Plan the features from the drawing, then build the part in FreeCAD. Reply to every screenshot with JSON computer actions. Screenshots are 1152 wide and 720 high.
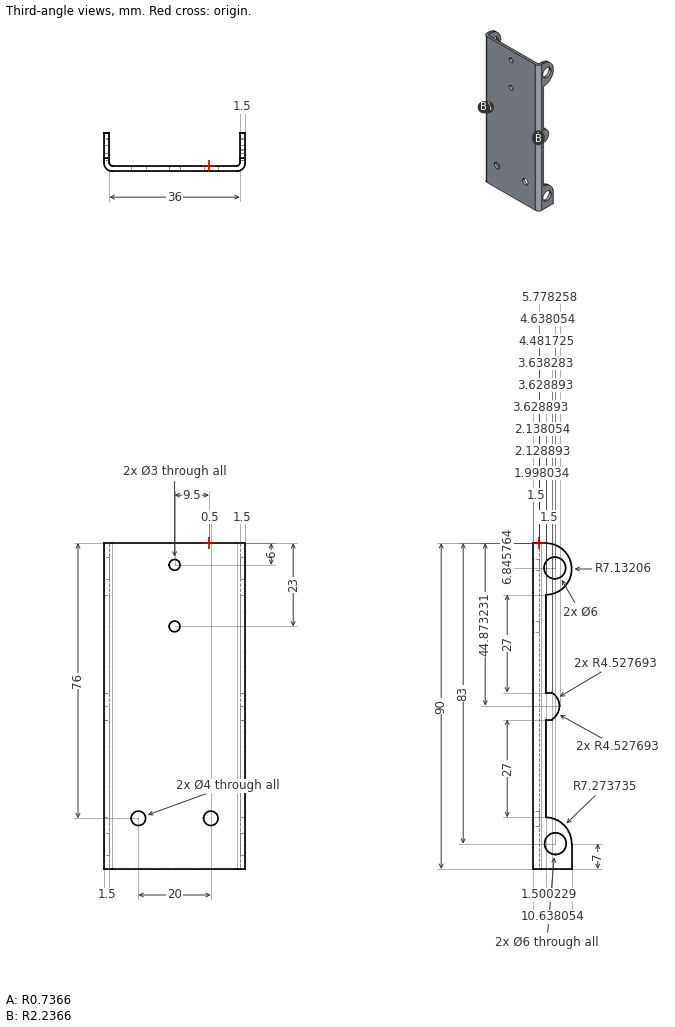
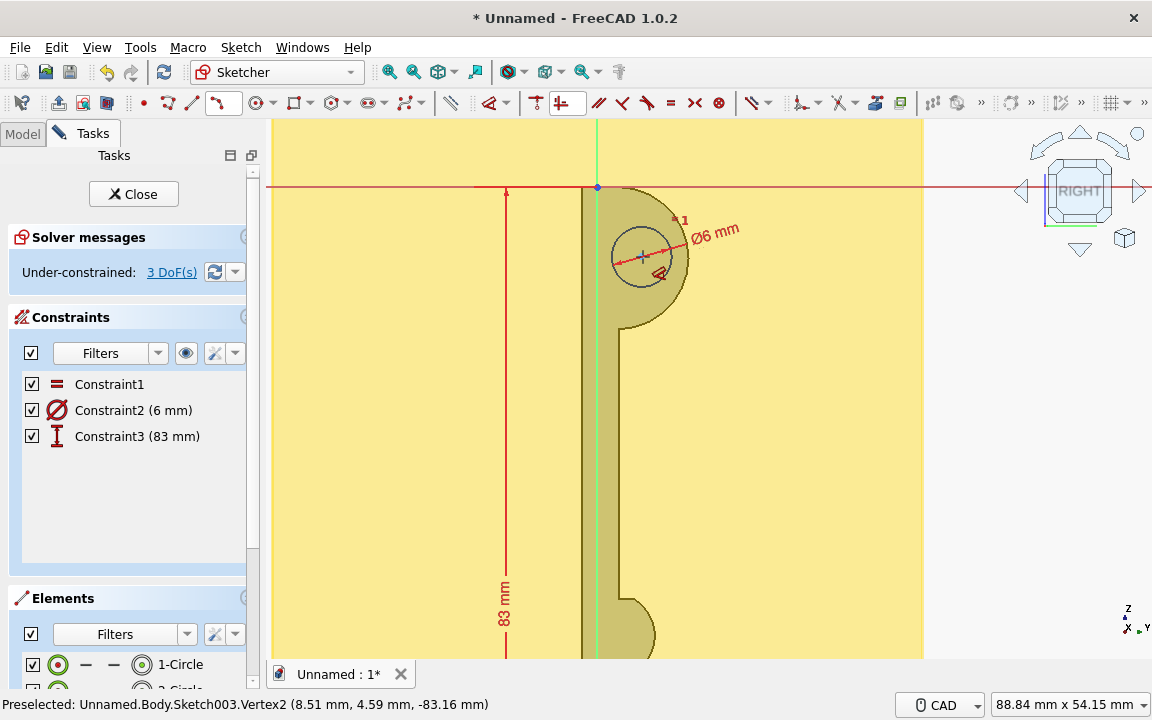
{"action": "left_click", "coordinate": [642, 257]}
{"action": "left_click", "coordinate": [620, 153]}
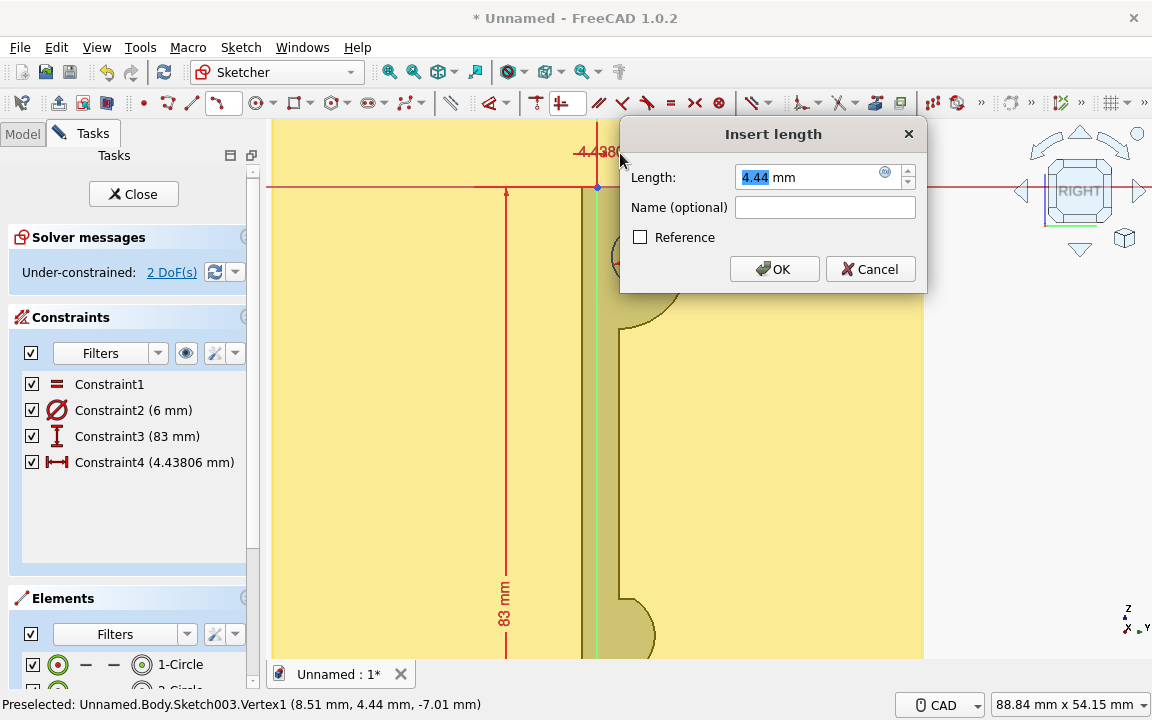
{"action": "type", "text": "4.481725"}
{"action": "key", "text": "Return"}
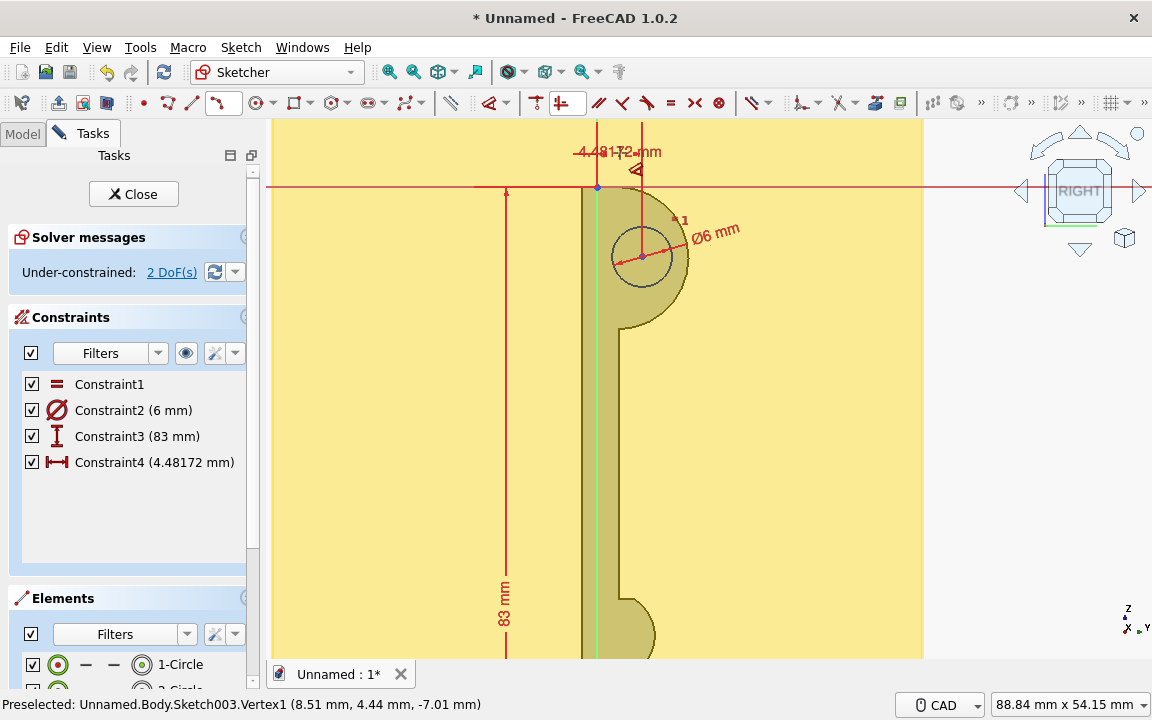
{"action": "left_click", "coordinate": [642, 257]}
{"action": "left_click", "coordinate": [563, 222]}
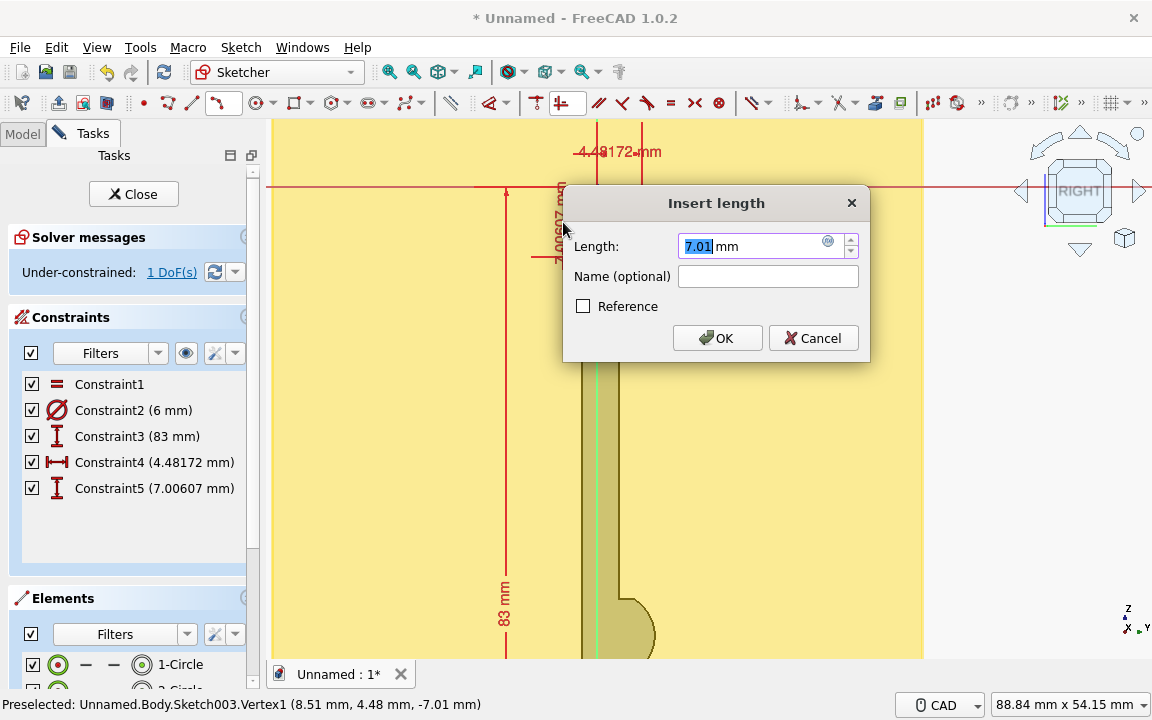
{"action": "type", "text": "6.845764"}
{"action": "key", "text": "Return"}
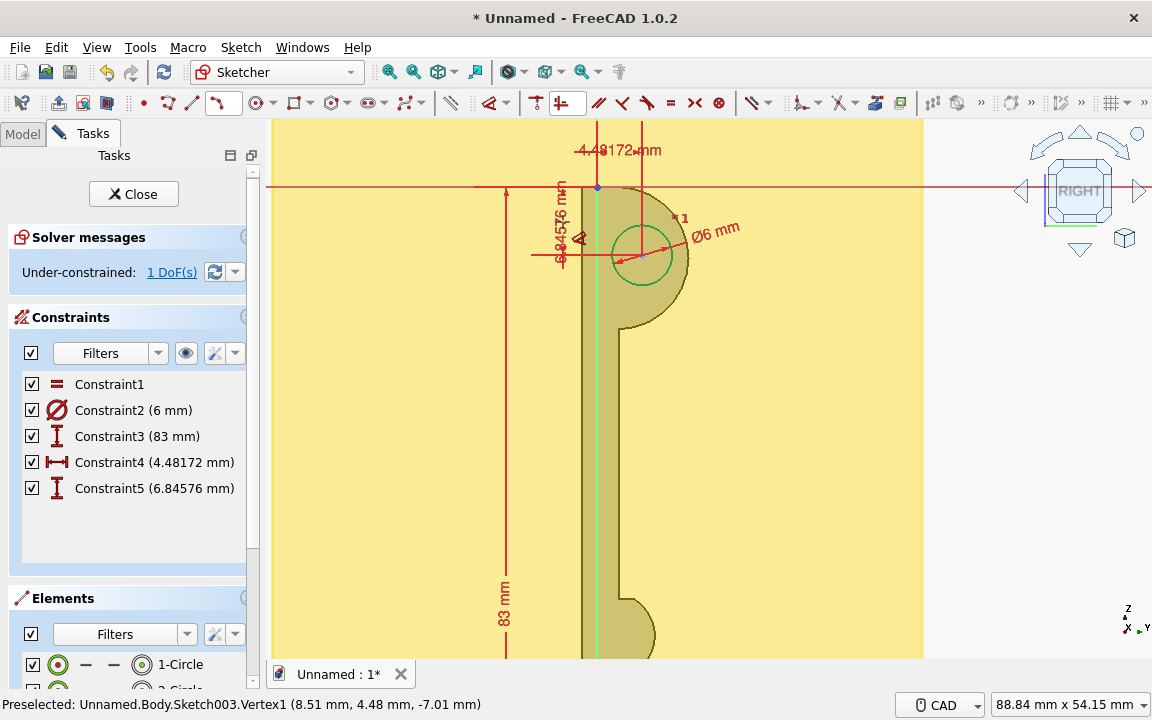
{"action": "scroll", "coordinate": [643, 257], "scroll_direction": "down", "scroll_amount": 5}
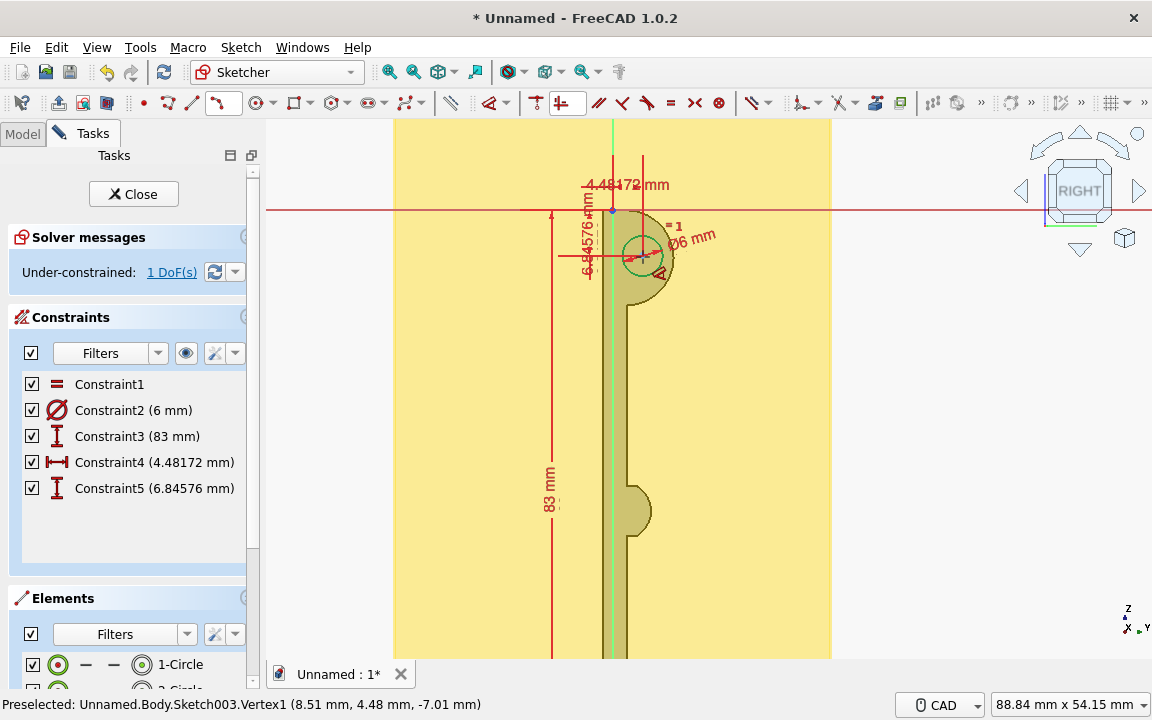
{"action": "scroll", "coordinate": [643, 536], "scroll_direction": "up", "scroll_amount": 5}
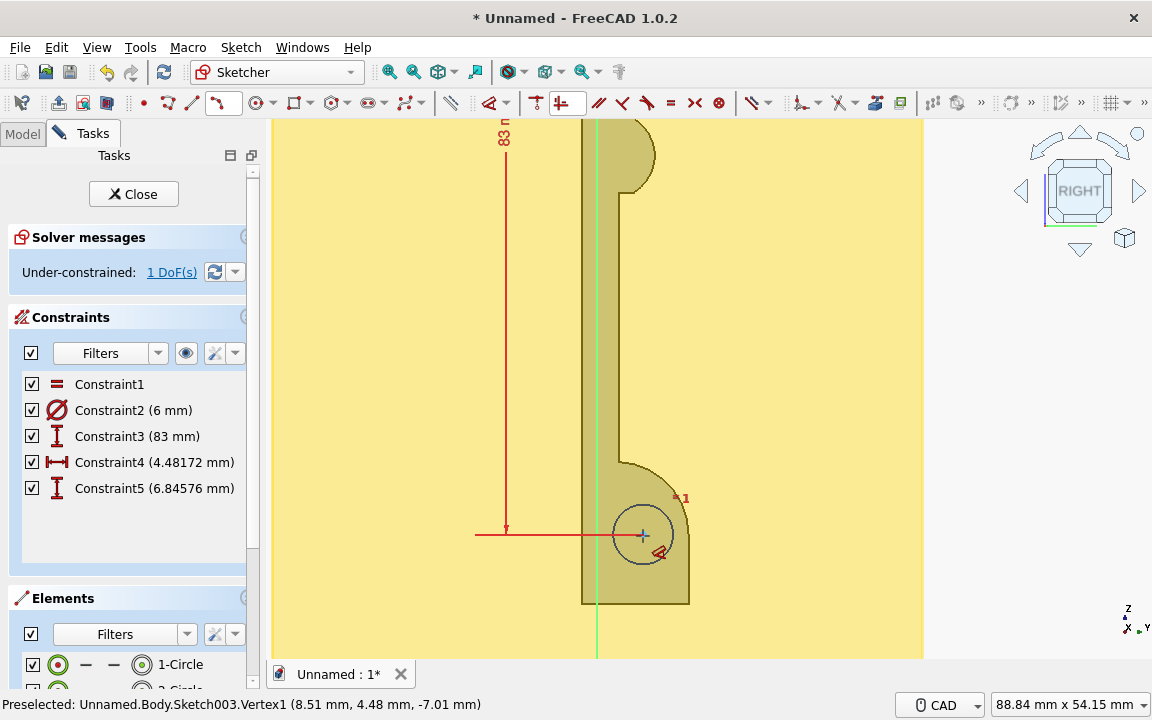
{"action": "left_click", "coordinate": [643, 535]}
{"action": "left_click", "coordinate": [620, 593]}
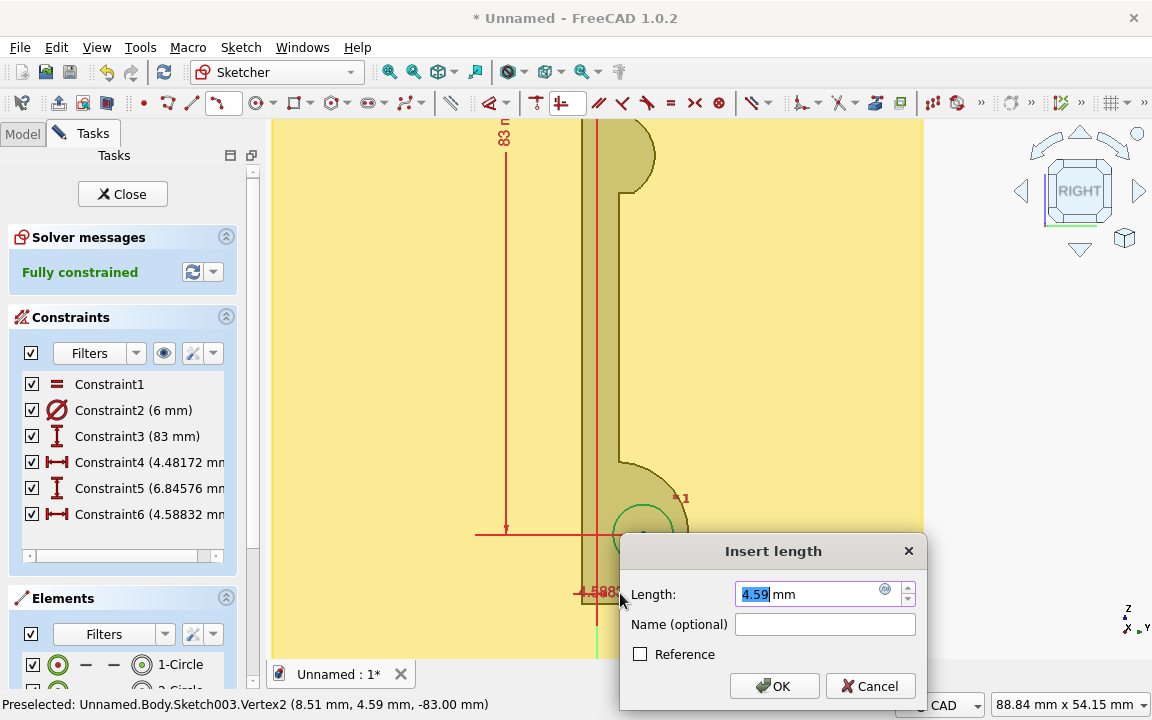
{"action": "type", "text": "4.638054"}
{"action": "key", "text": "Return"}
{"action": "key", "text": "Escape"}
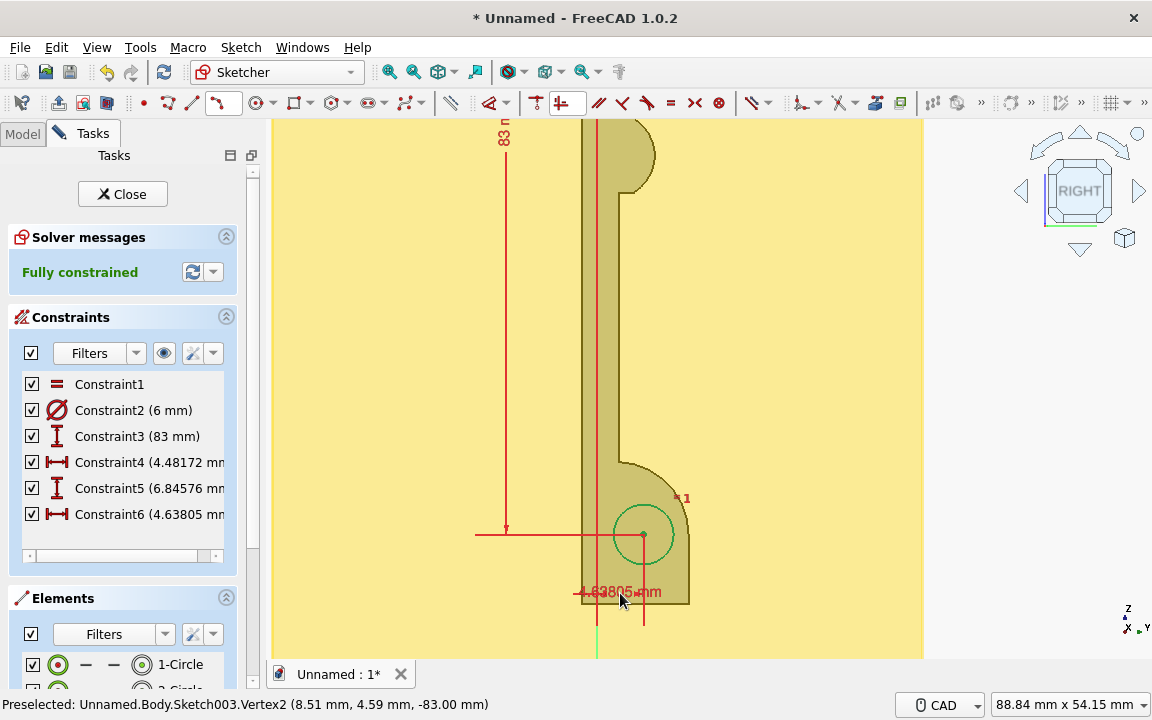
{"action": "left_click", "coordinate": [123, 194]}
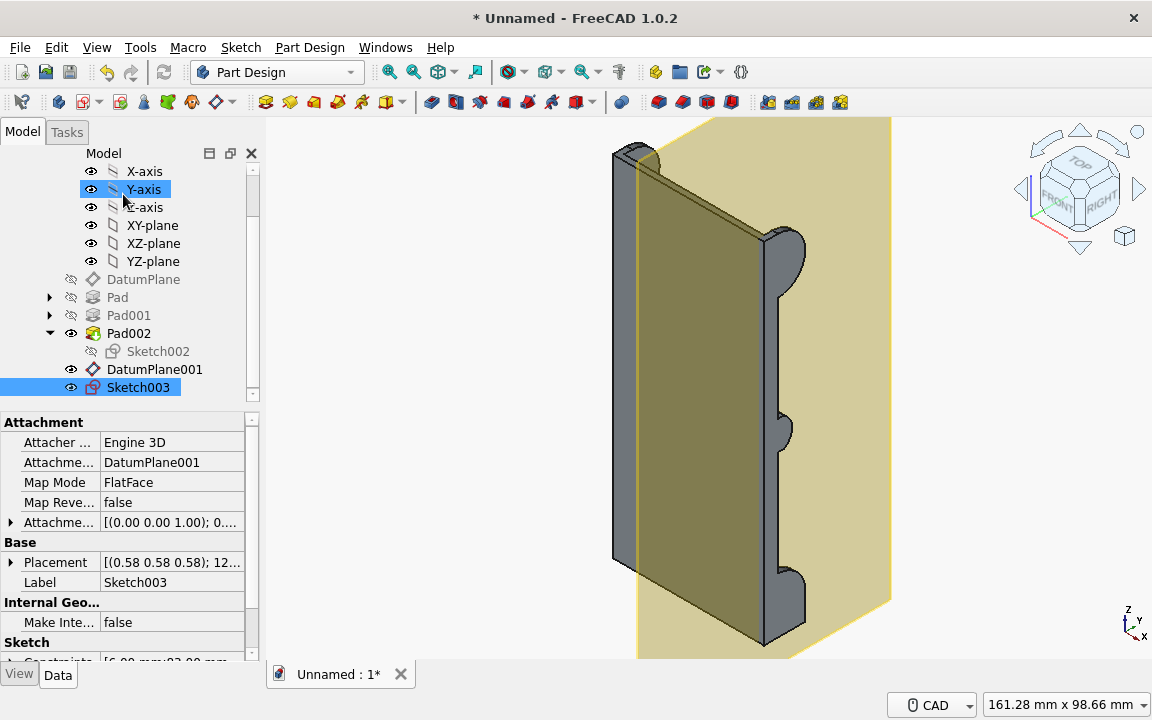
{"action": "left_click", "coordinate": [432, 102]}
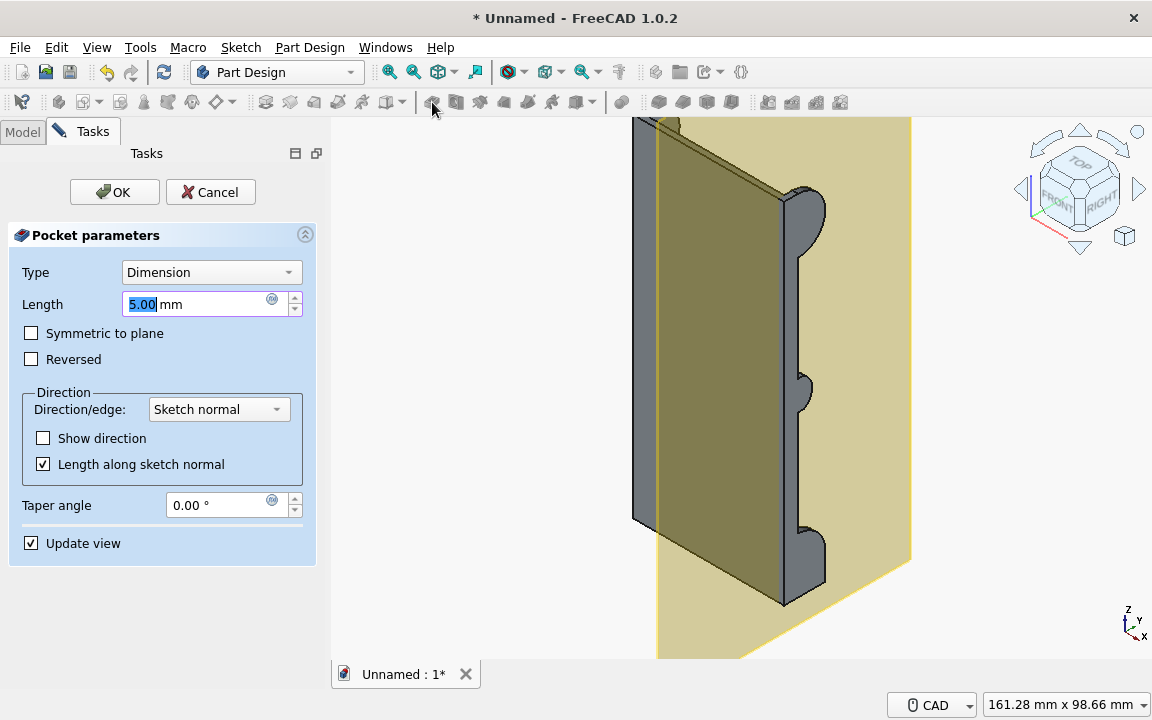
{"action": "type", "text": "1.5"}
{"action": "key", "text": "Tab"}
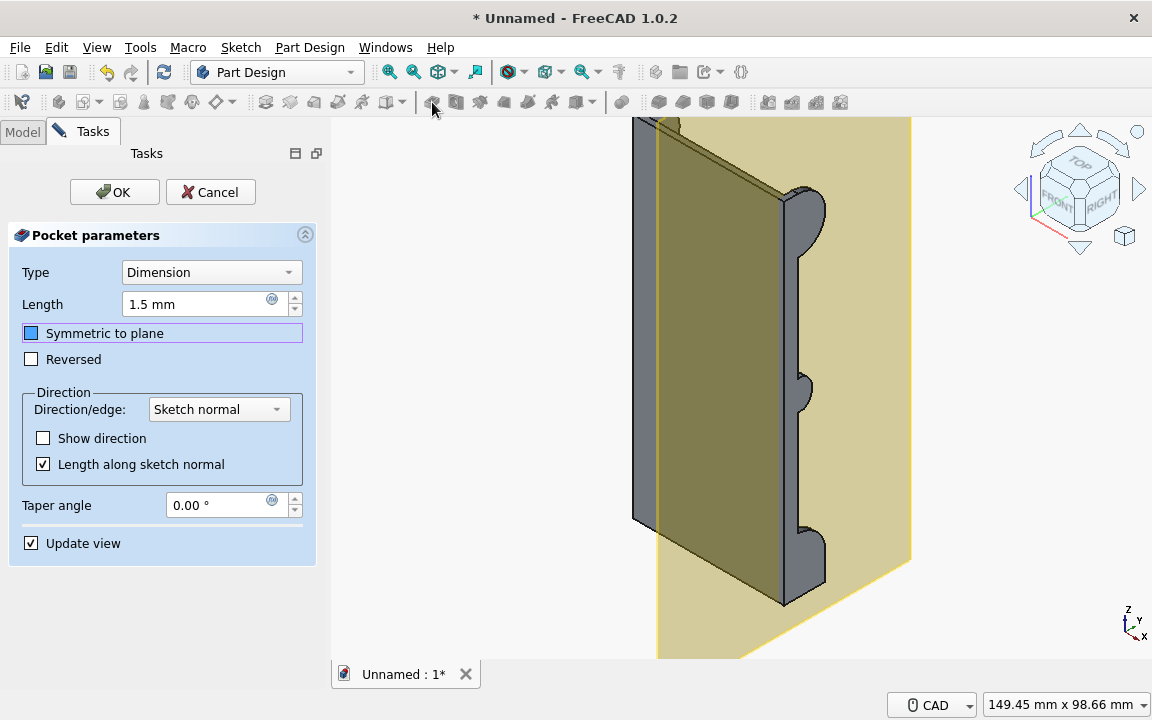
{"action": "left_click", "coordinate": [30, 359]}